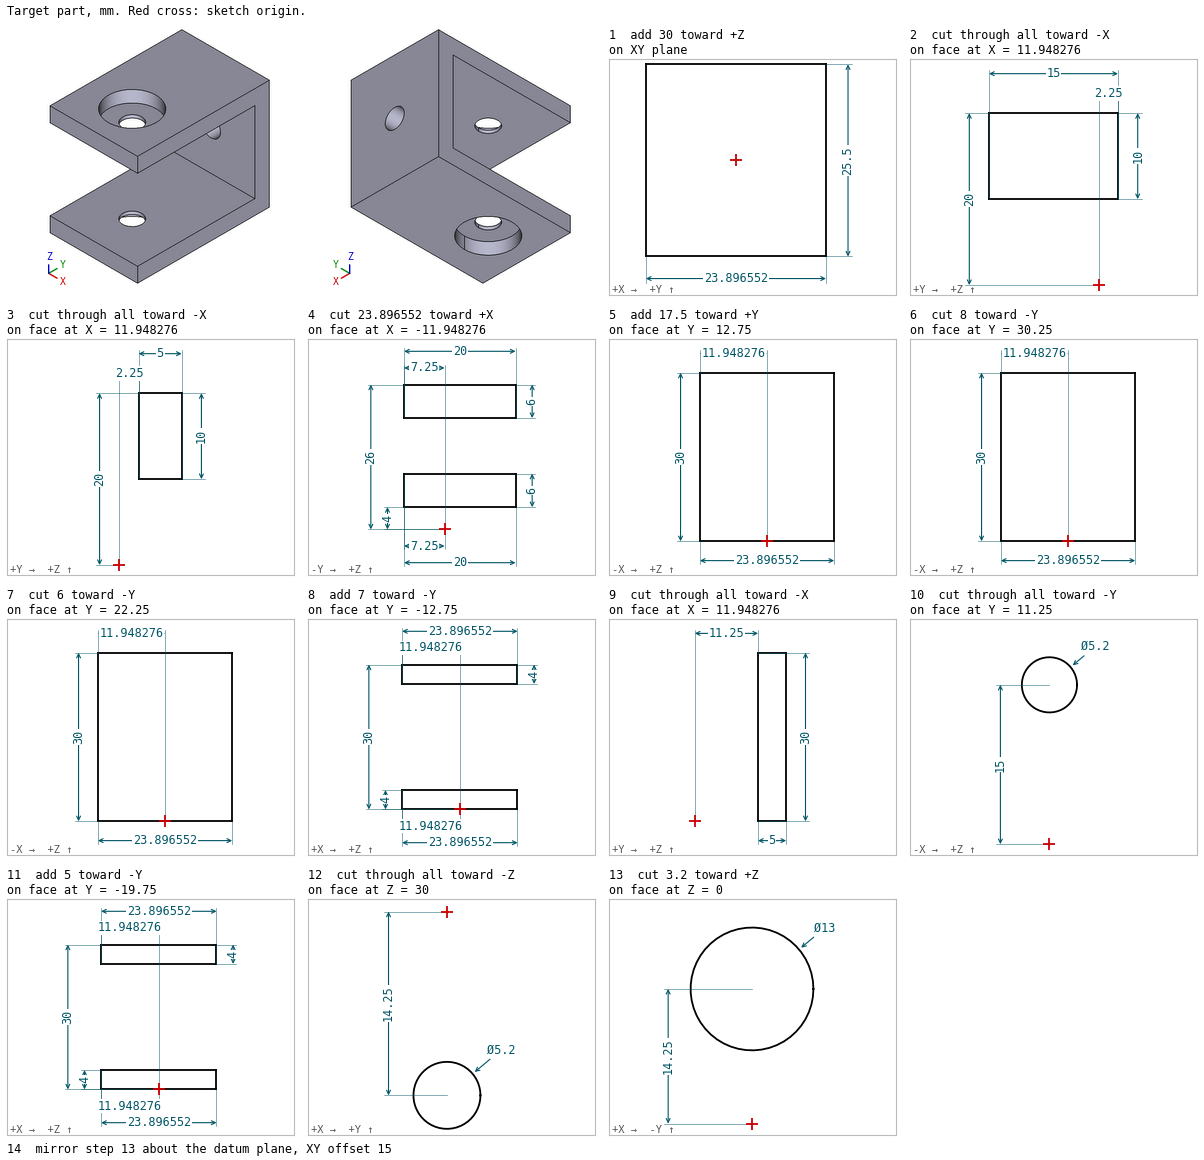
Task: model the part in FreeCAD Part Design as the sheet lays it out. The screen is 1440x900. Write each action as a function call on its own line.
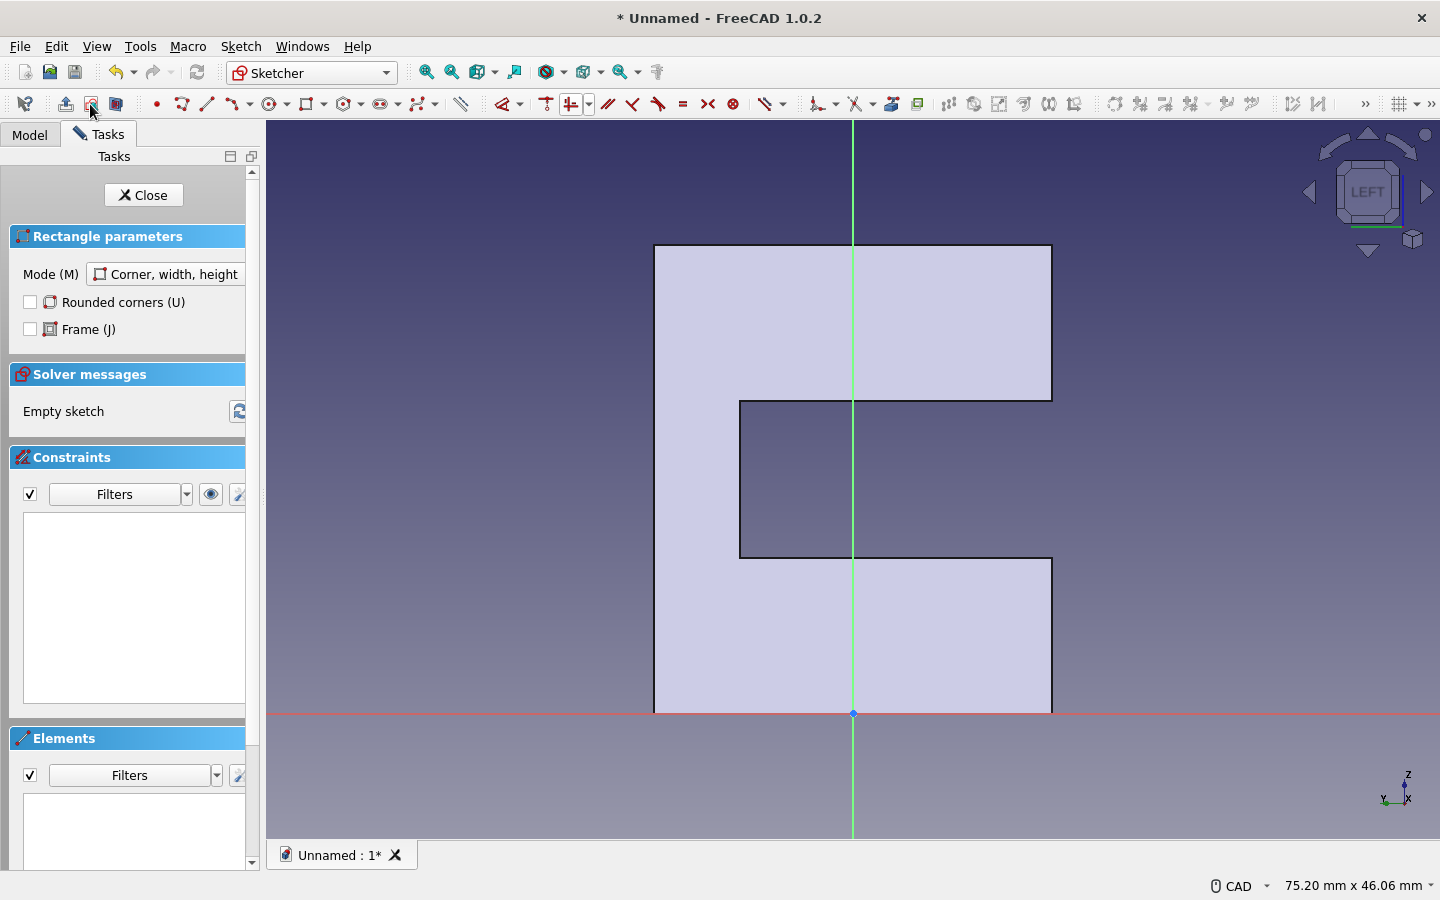
click(740, 558)
move(1052, 651)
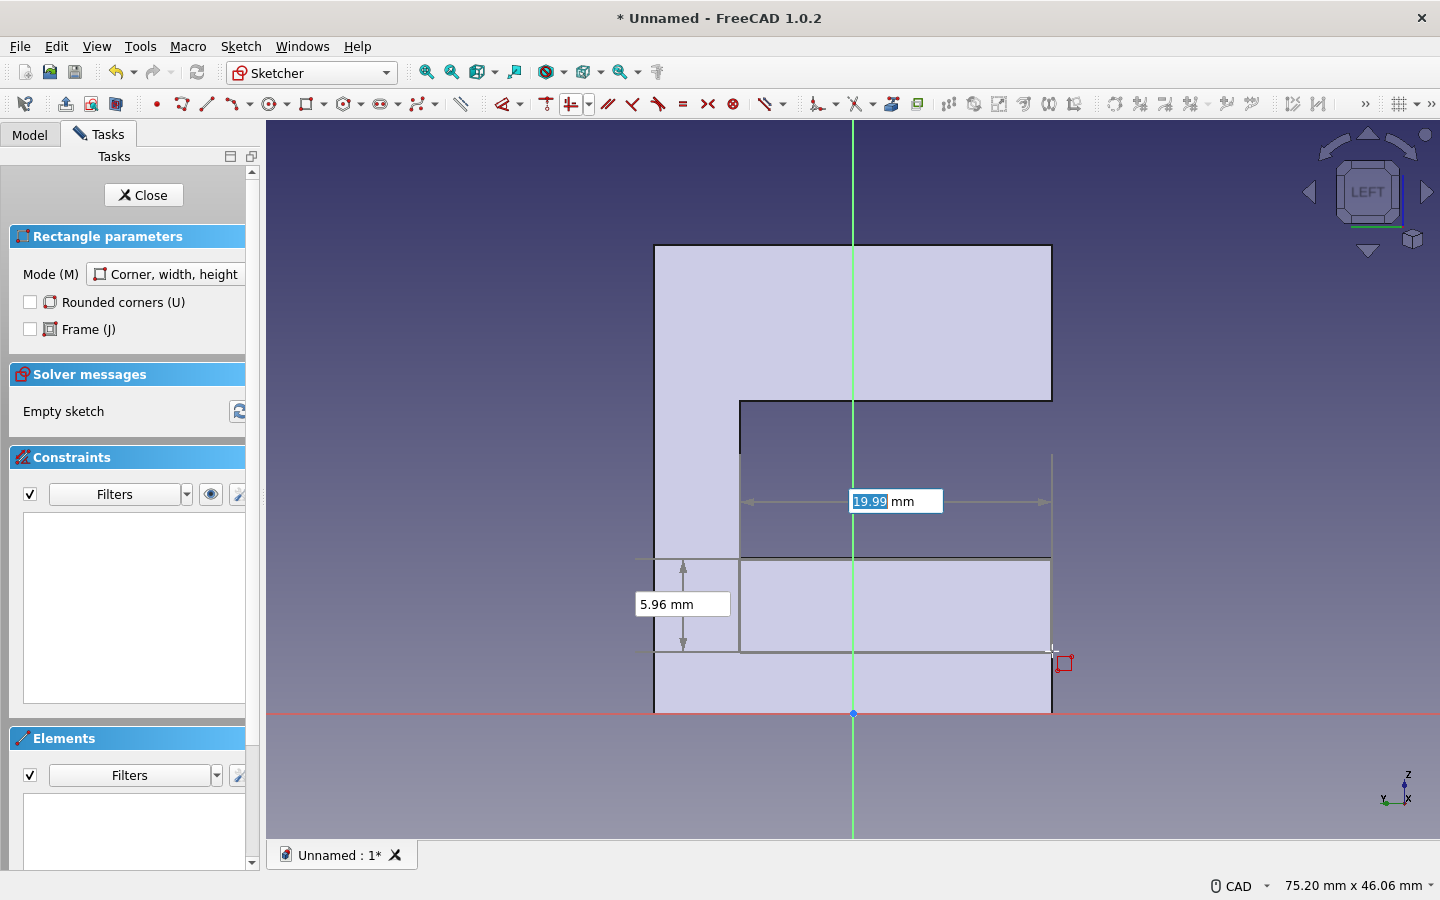
text(20)
key(Tab)
text(6)
key(Return)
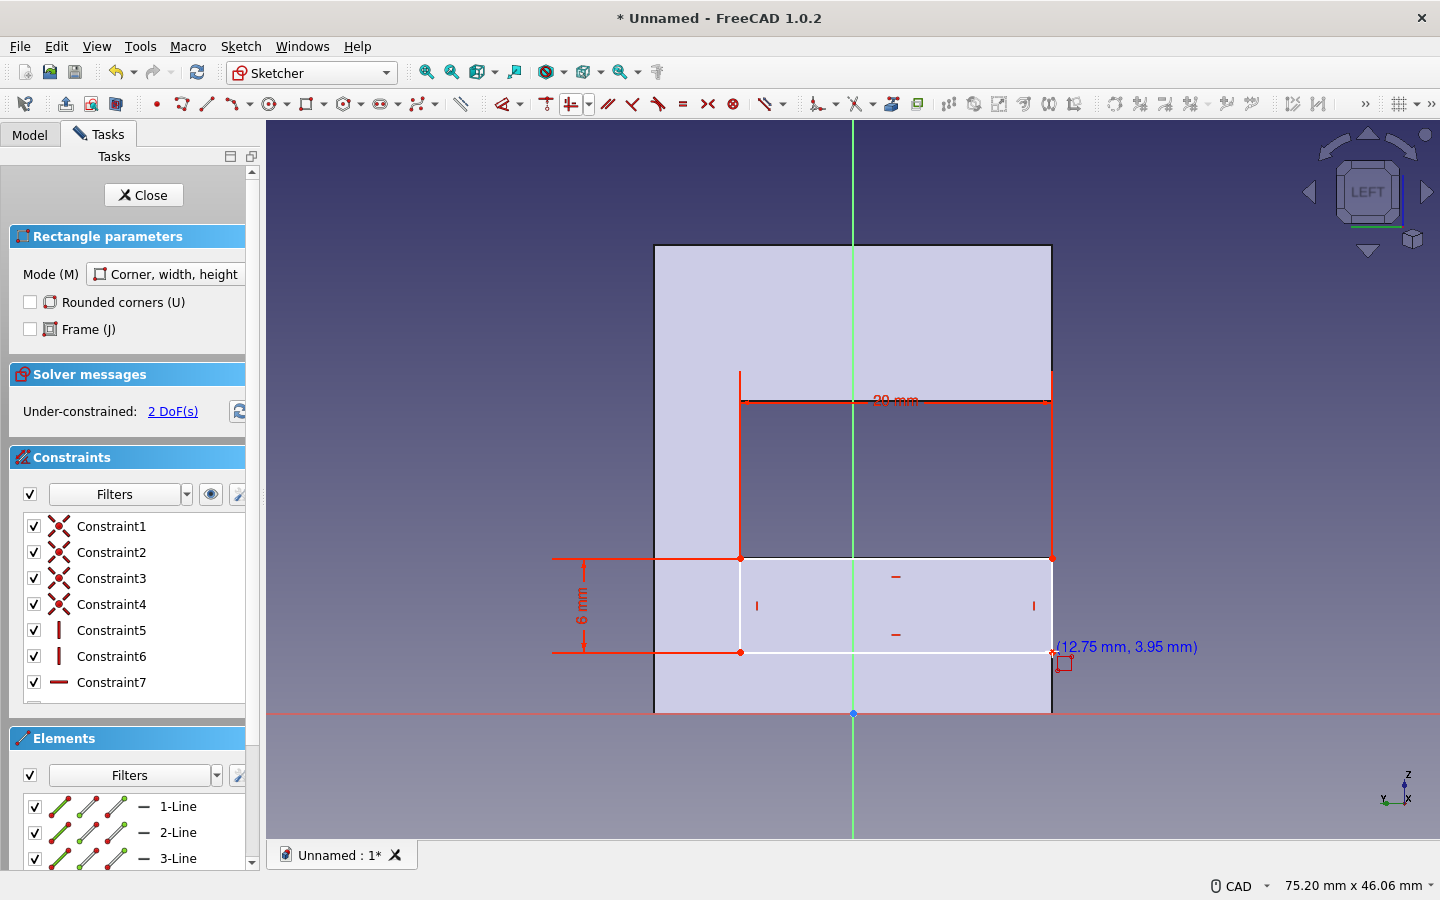
click(740, 308)
move(1052, 401)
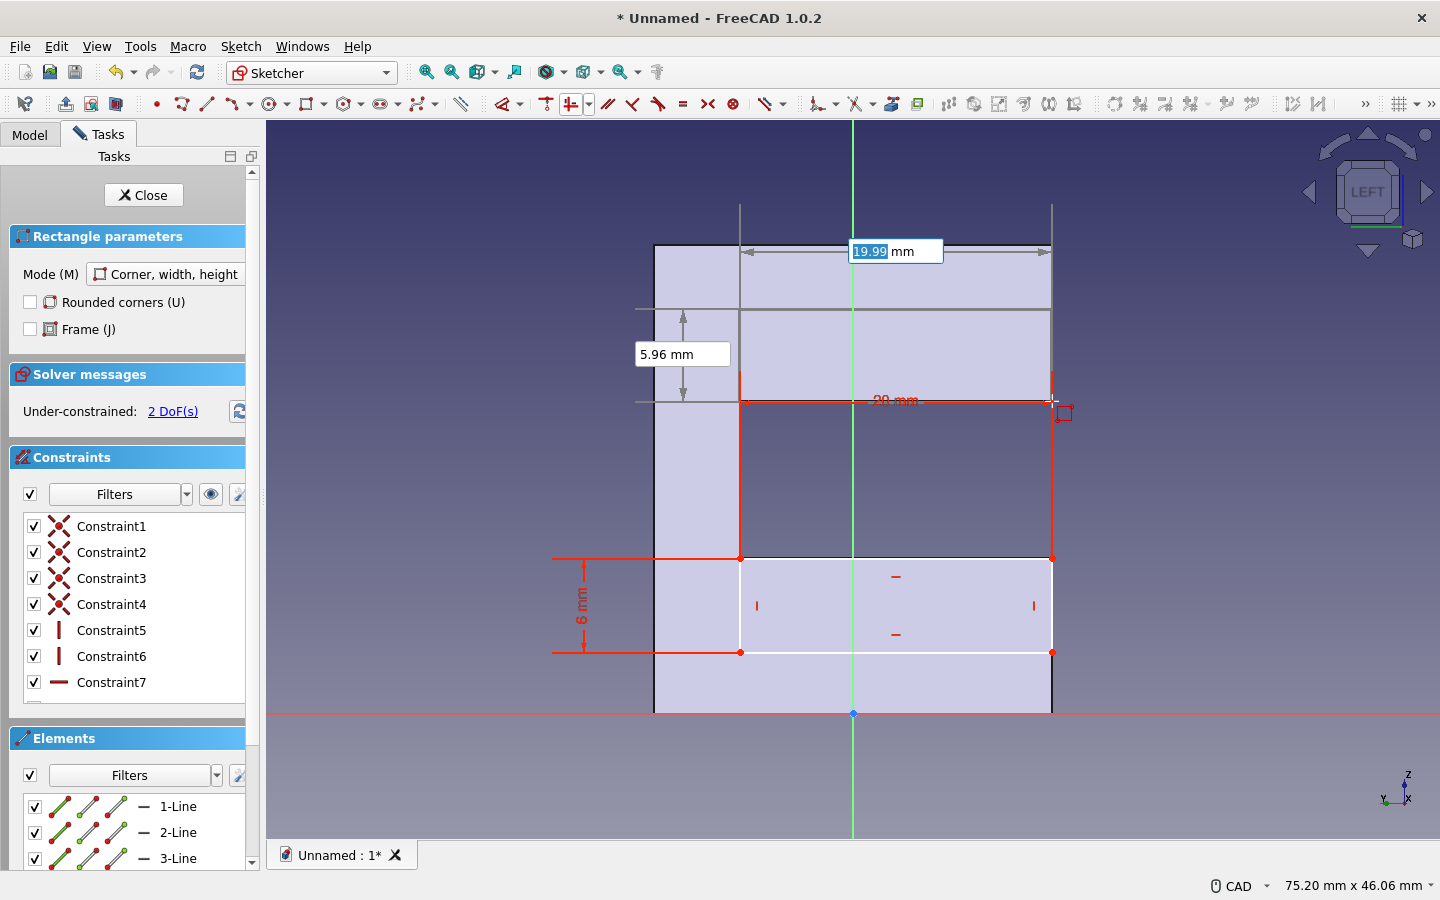
text(20)
key(Tab)
text(6)
key(Return)
key(Escape)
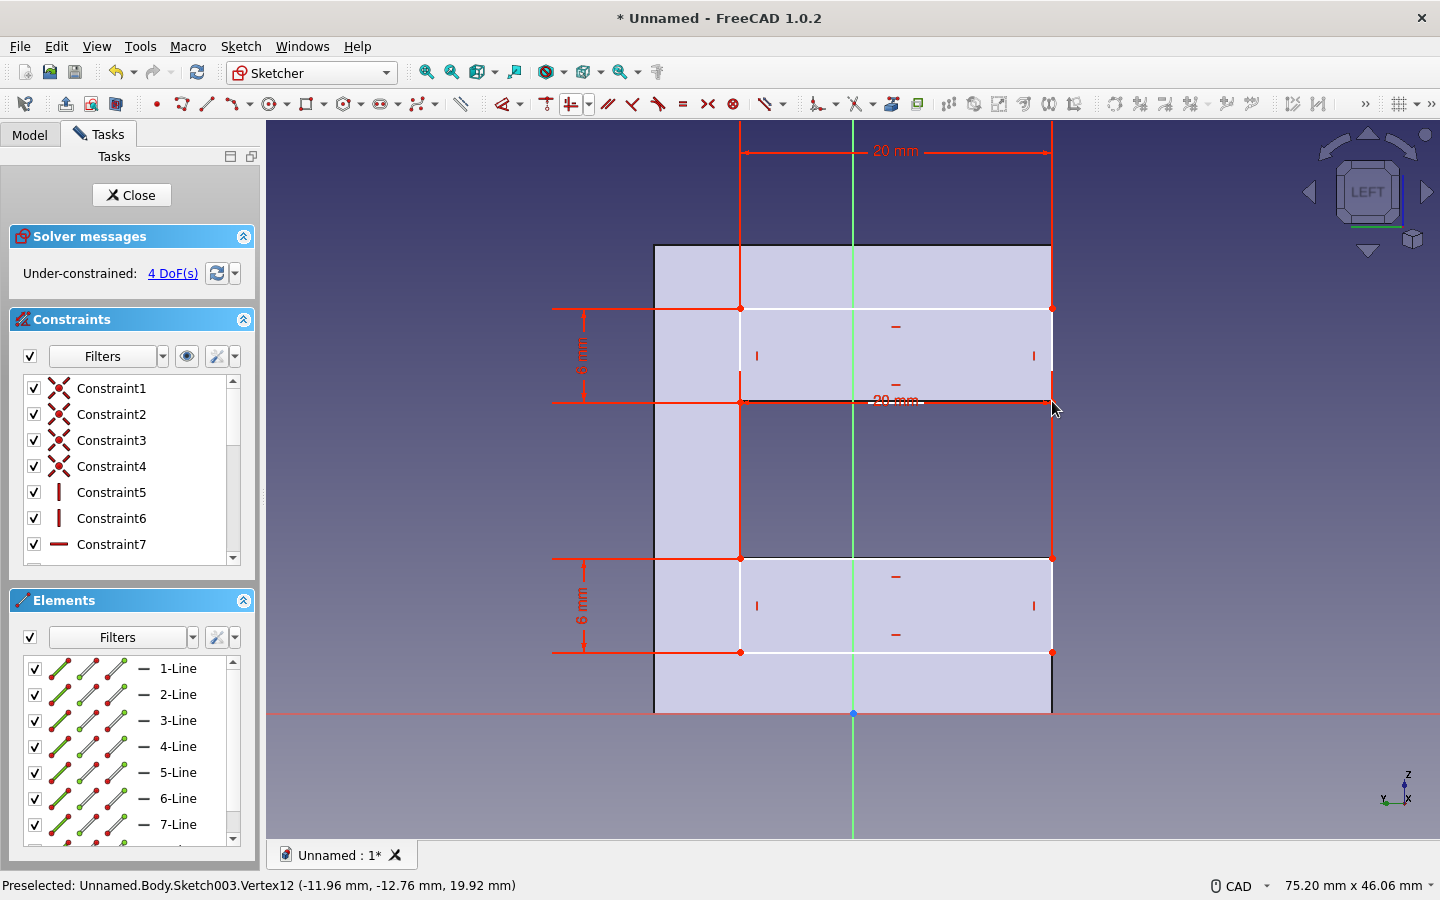
key(d)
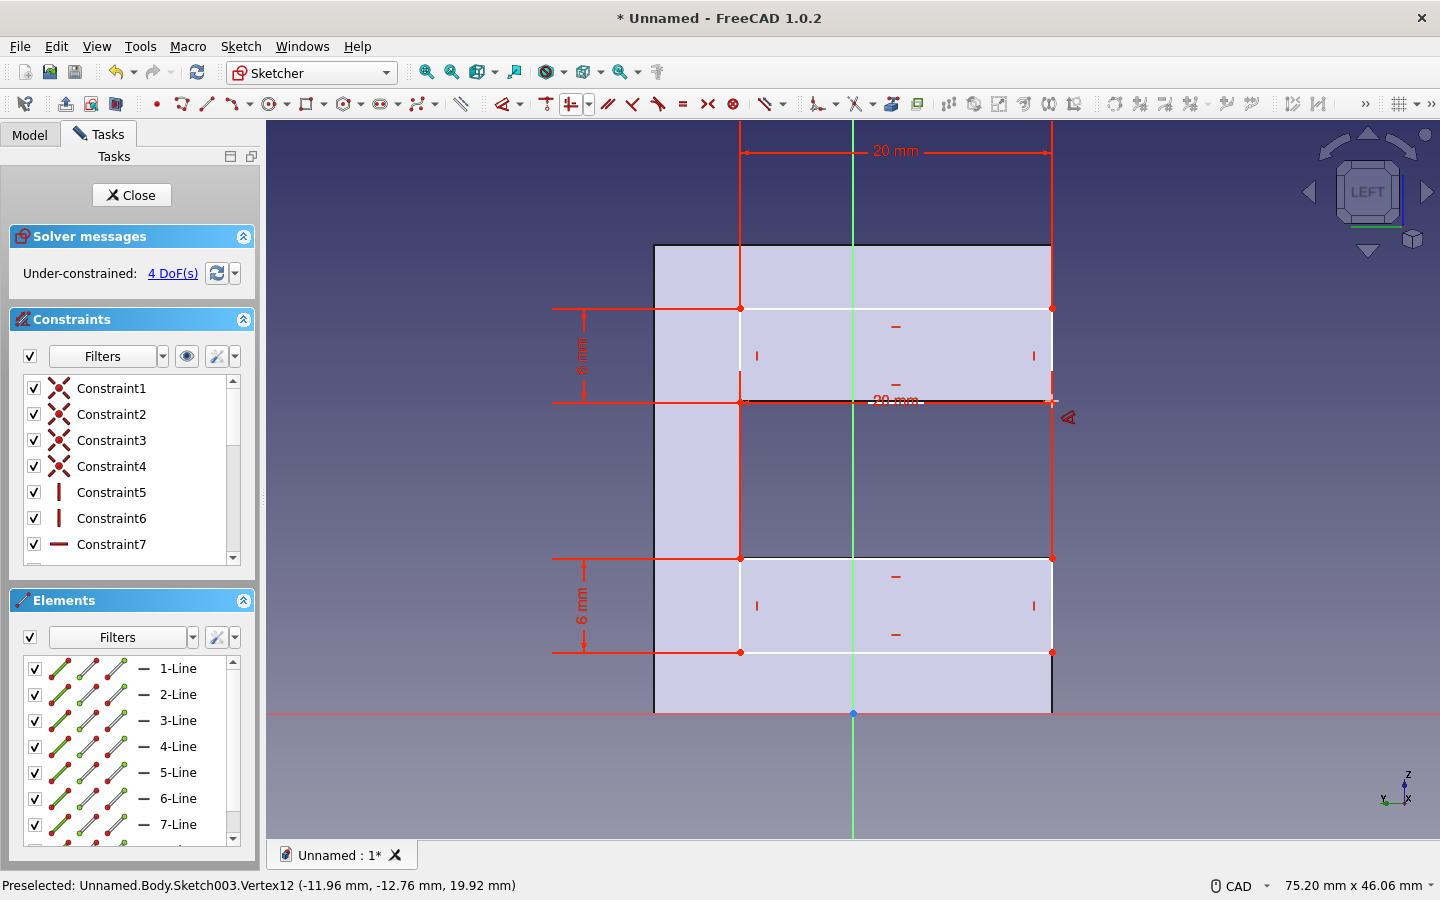
click(740, 653)
click(706, 683)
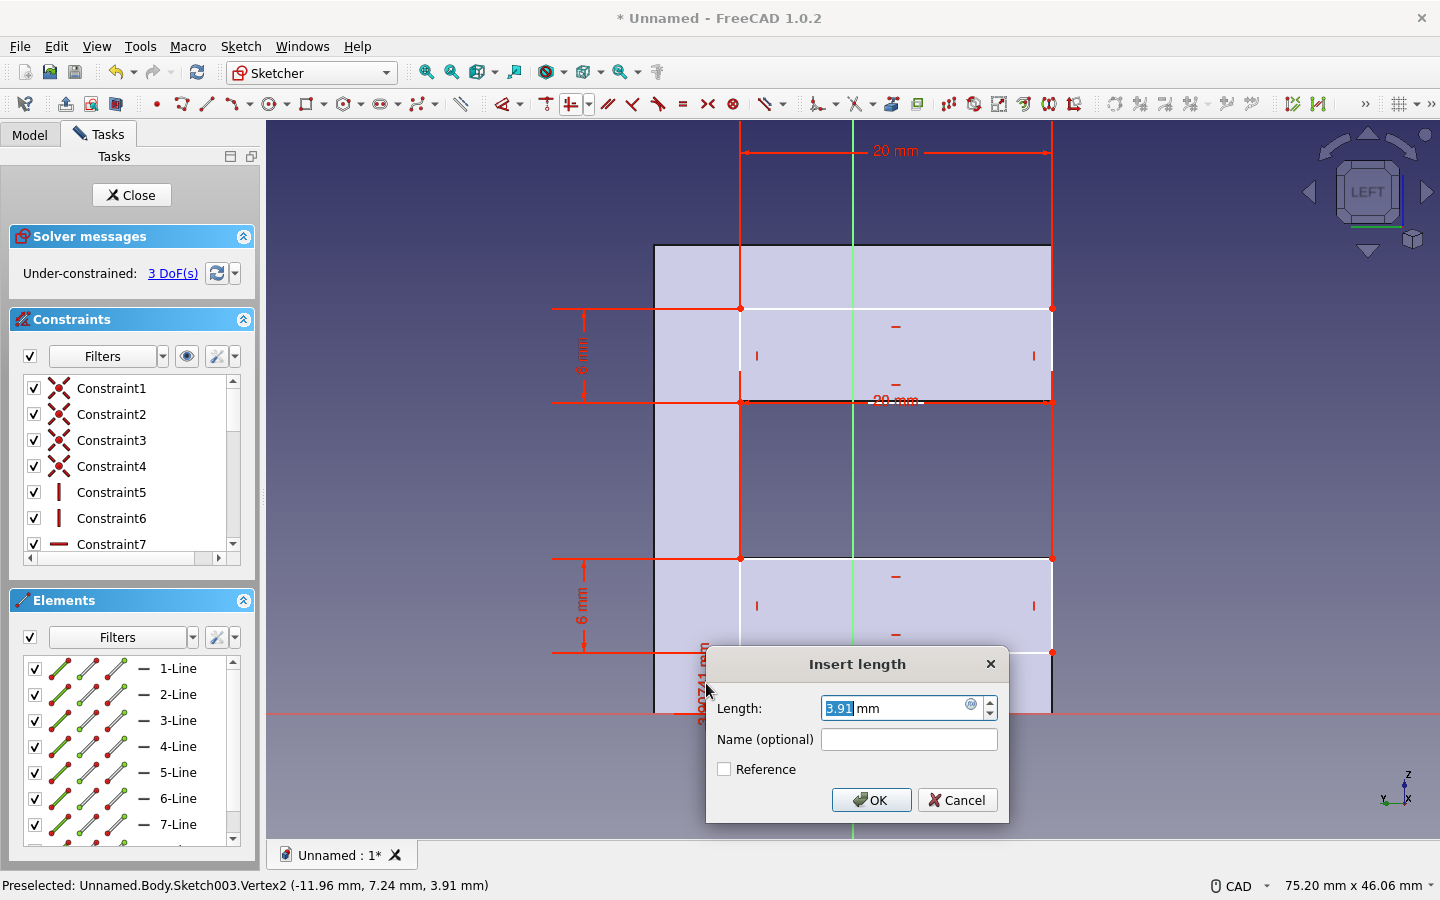
text(4)
key(Return)